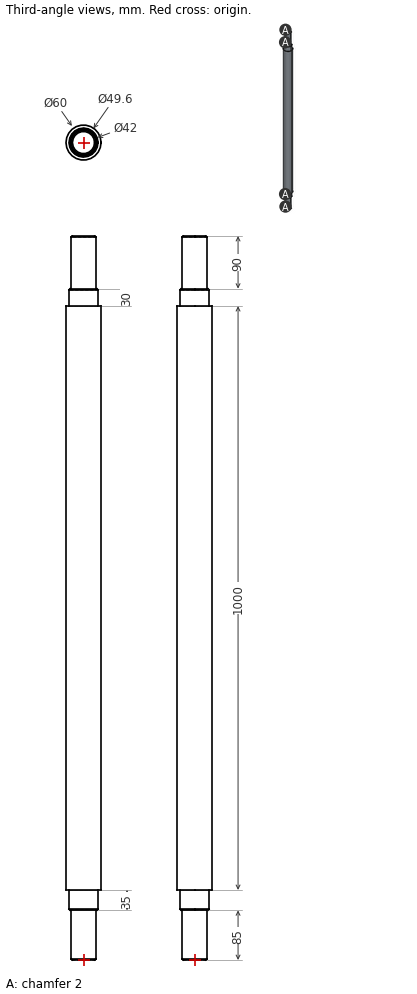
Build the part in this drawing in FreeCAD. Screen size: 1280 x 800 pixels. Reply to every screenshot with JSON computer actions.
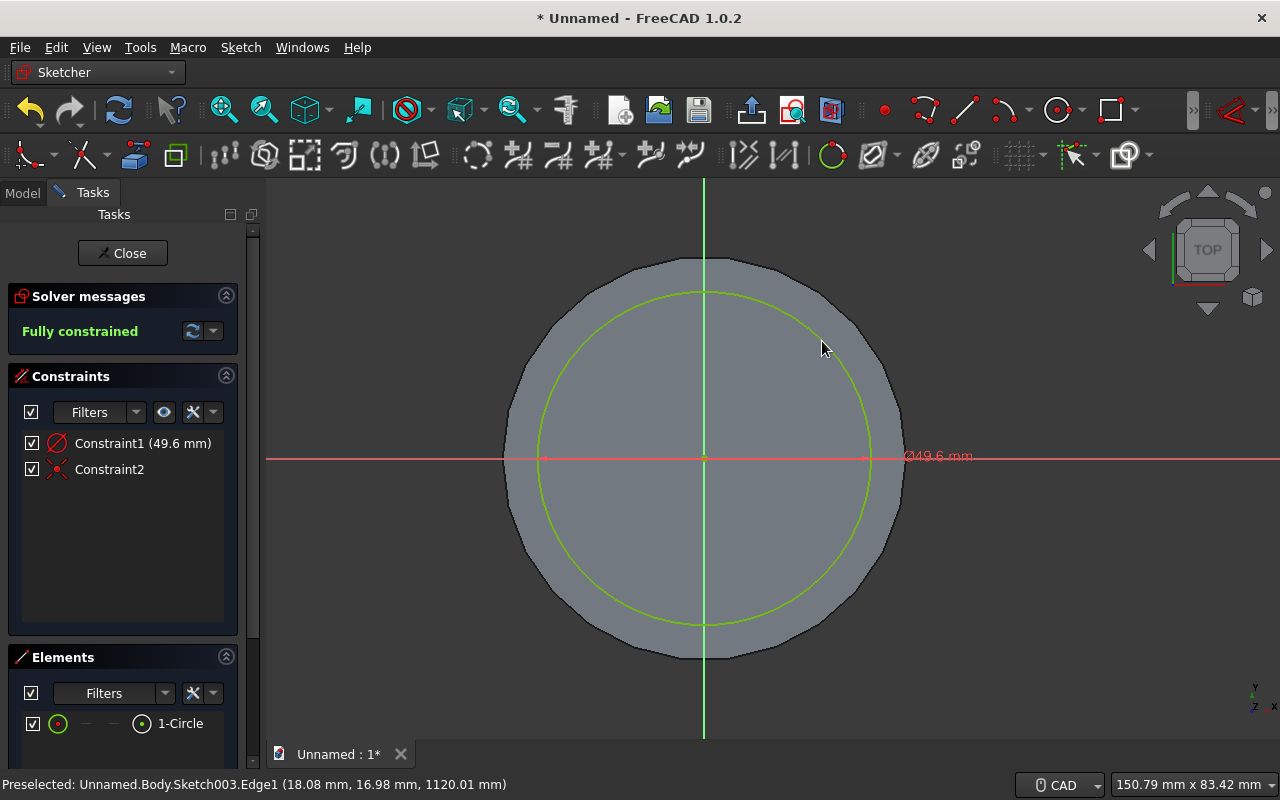
{"action": "left_click", "coordinate": [123, 253]}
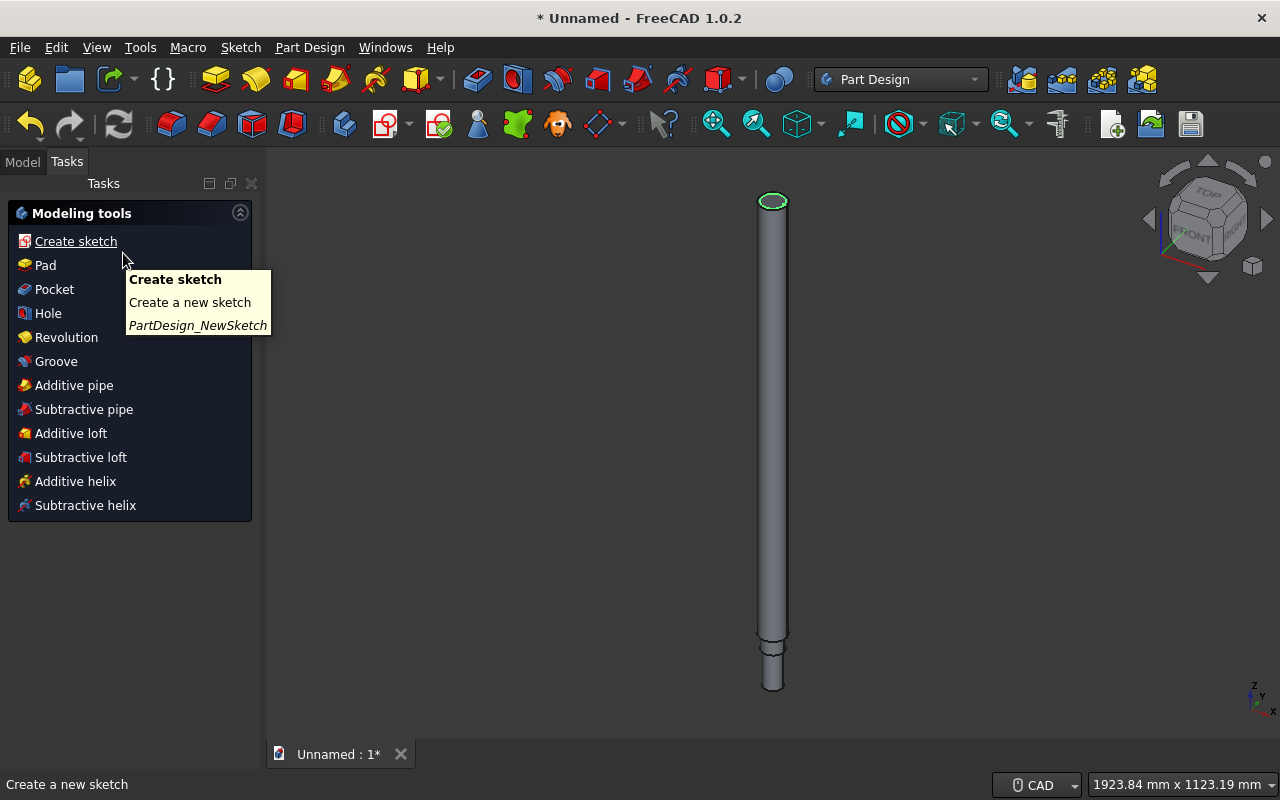
{"action": "left_click", "coordinate": [216, 80]}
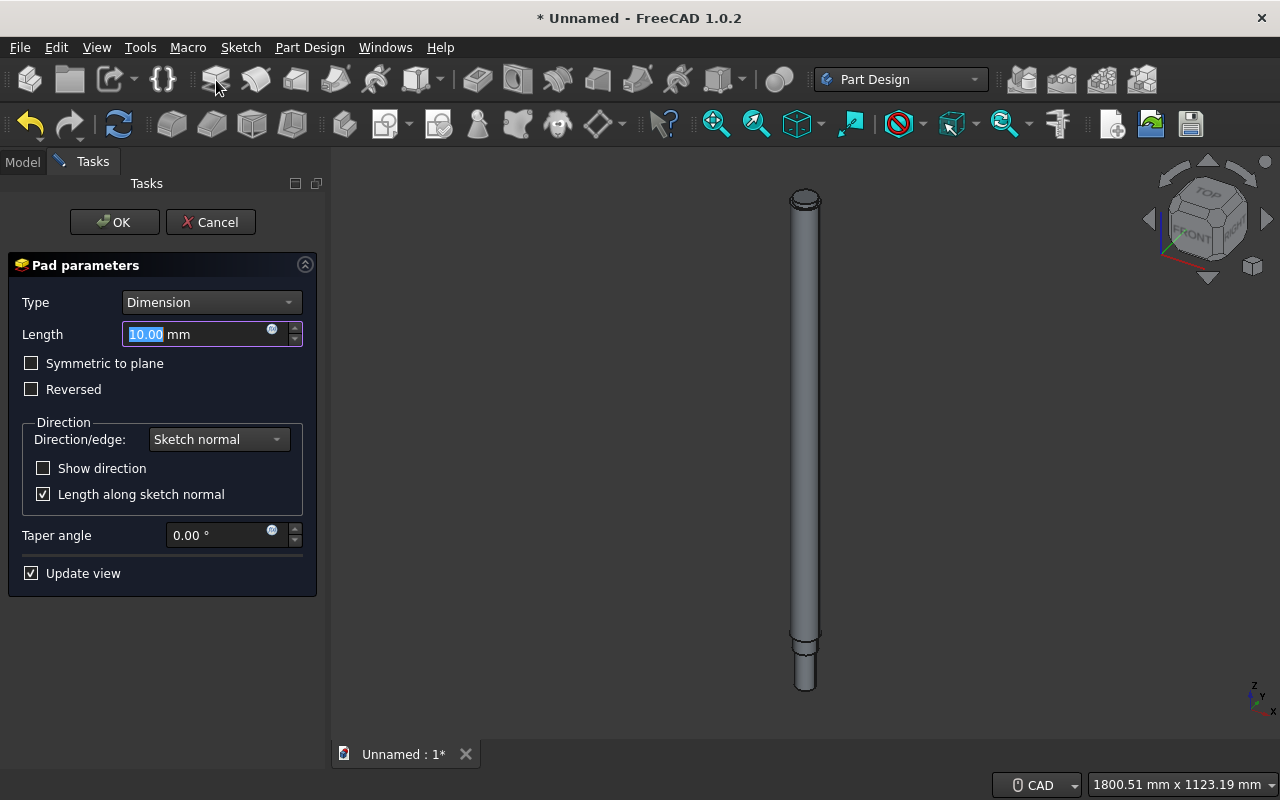
{"action": "type", "text": "30"}
{"action": "key", "text": "Tab"}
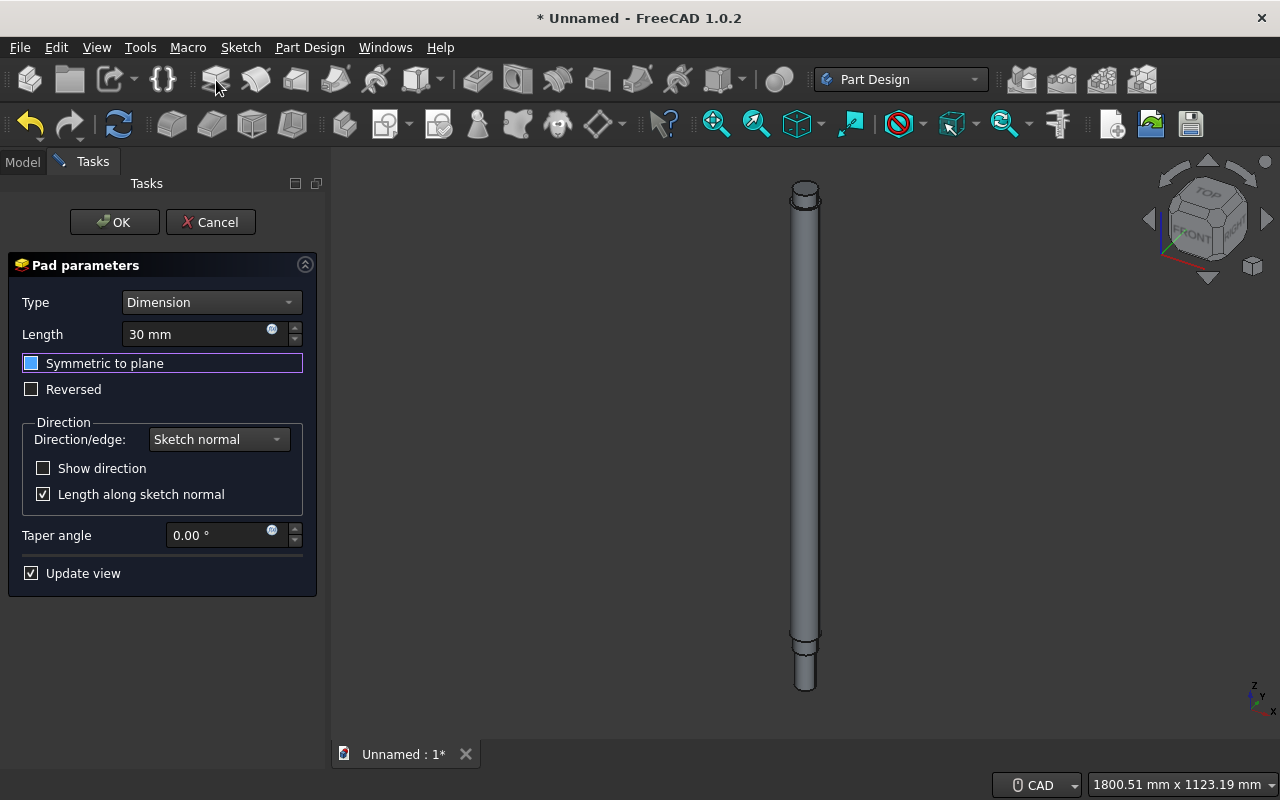
{"action": "left_click", "coordinate": [115, 222]}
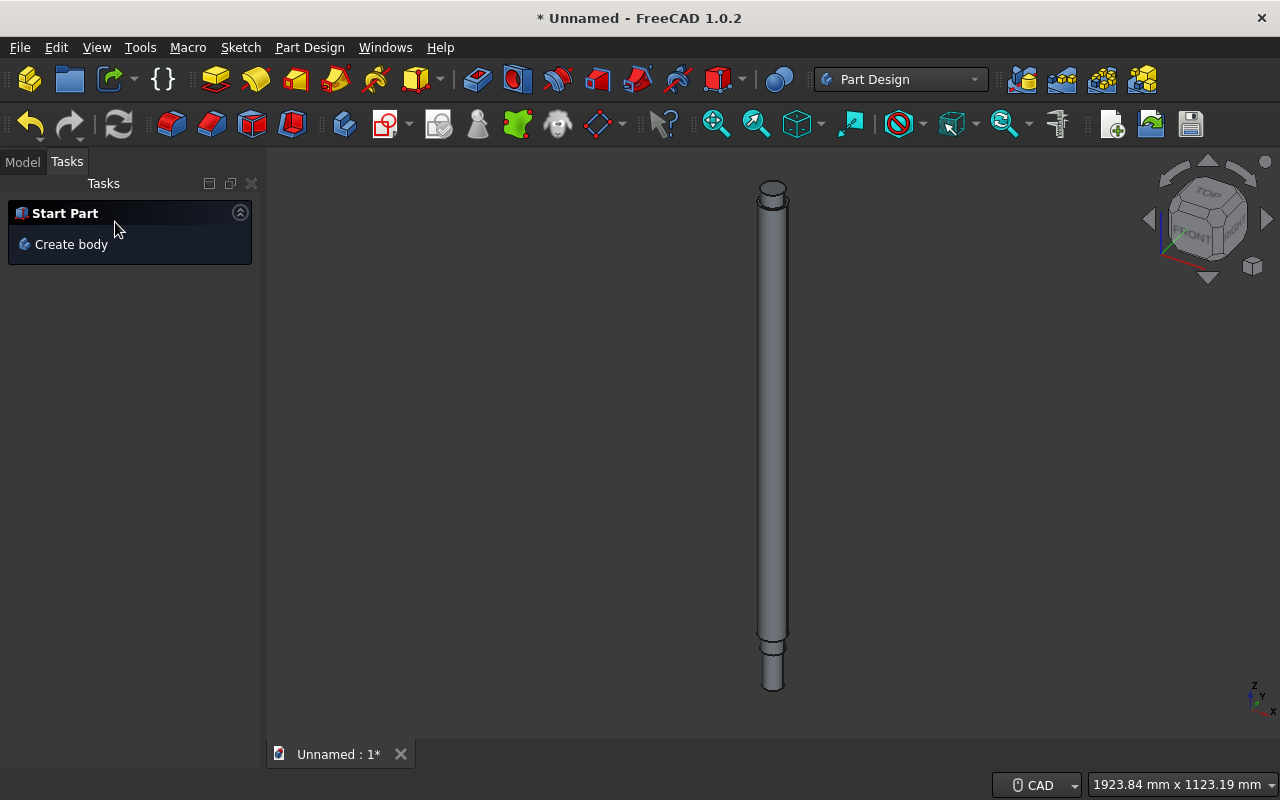
{"action": "left_click", "coordinate": [775, 185]}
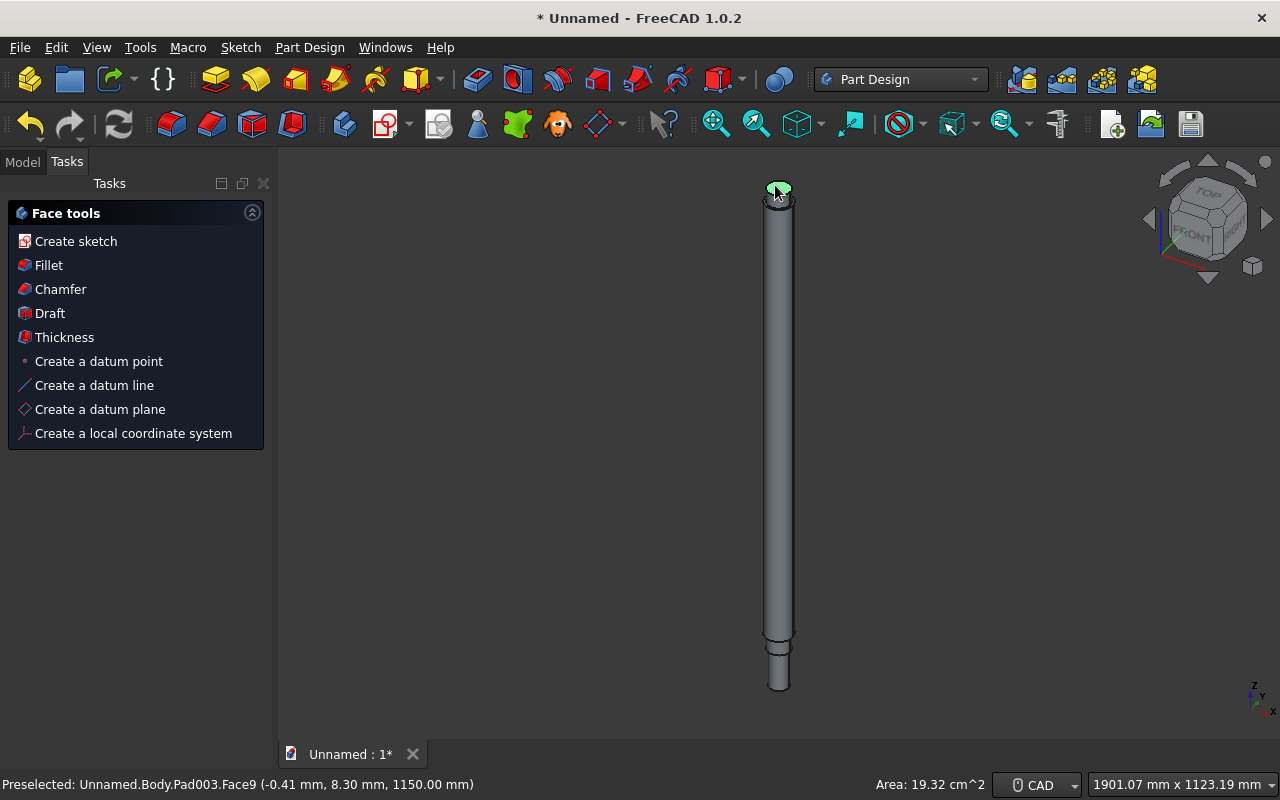
{"action": "left_click", "coordinate": [386, 124]}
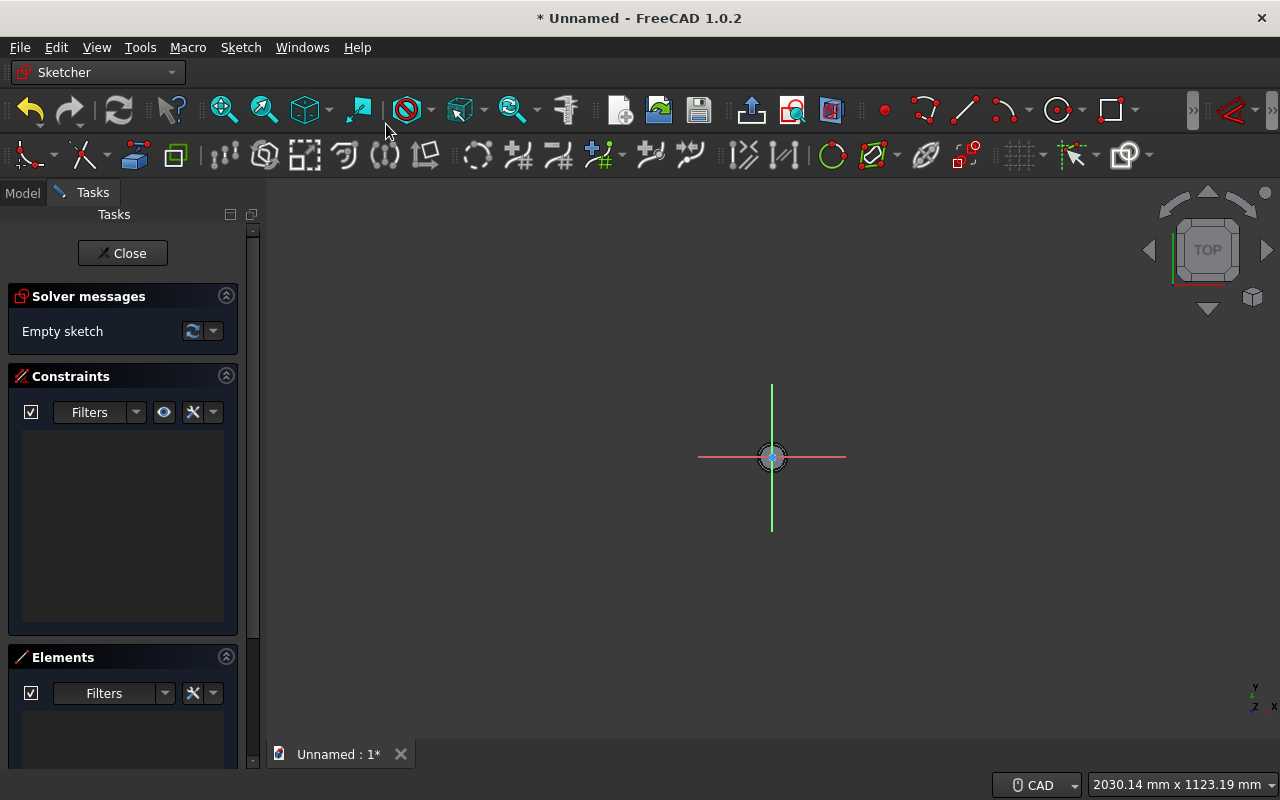
{"action": "scroll", "coordinate": [777, 457], "scroll_direction": "up", "scroll_amount": 14}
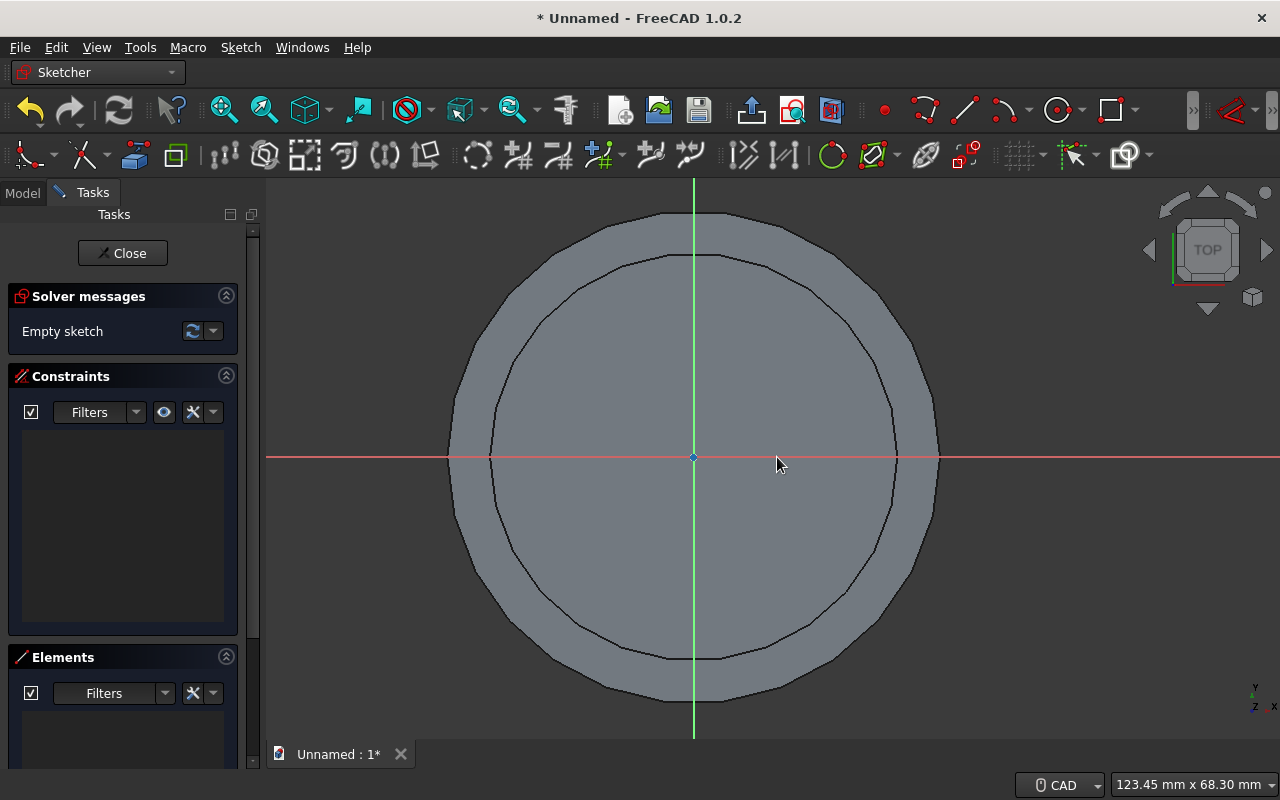
{"action": "key", "text": "g c"}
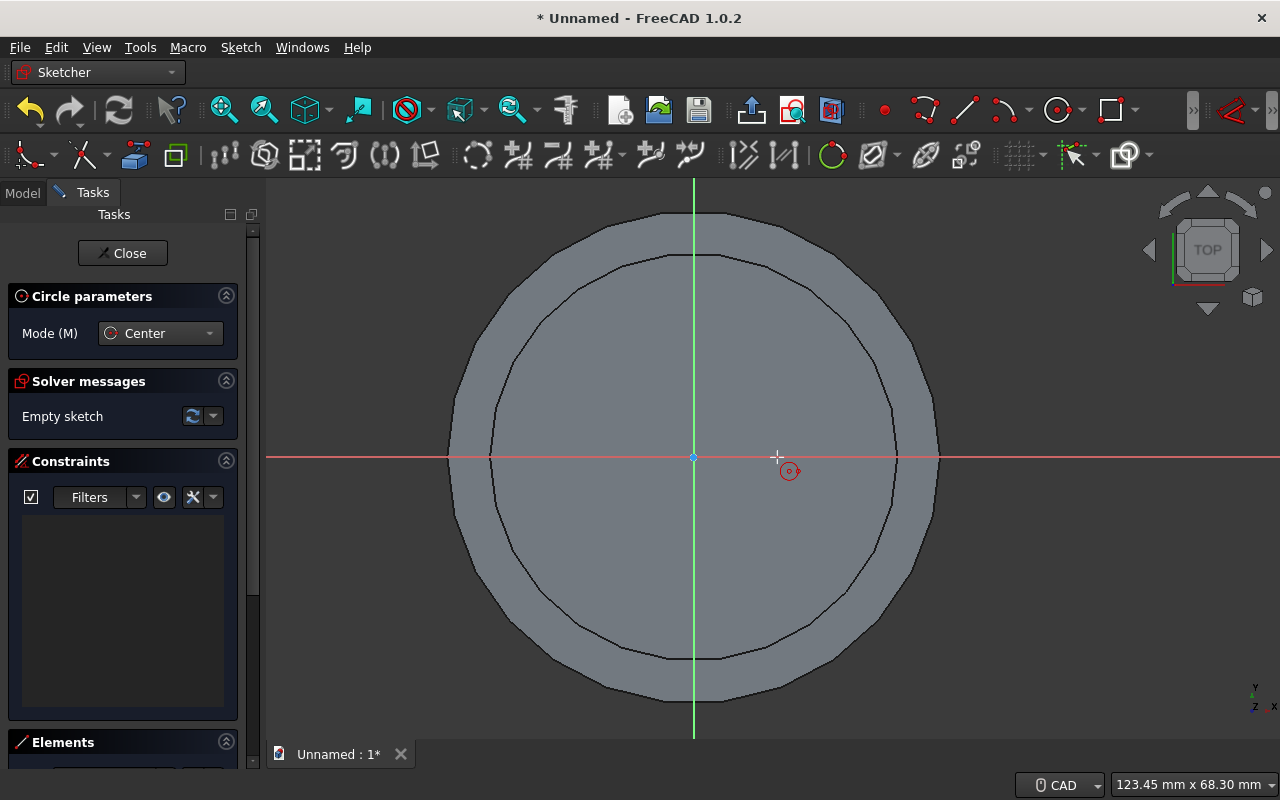
{"action": "left_click", "coordinate": [694, 457]}
{"action": "mouse_move", "coordinate": [816, 335]}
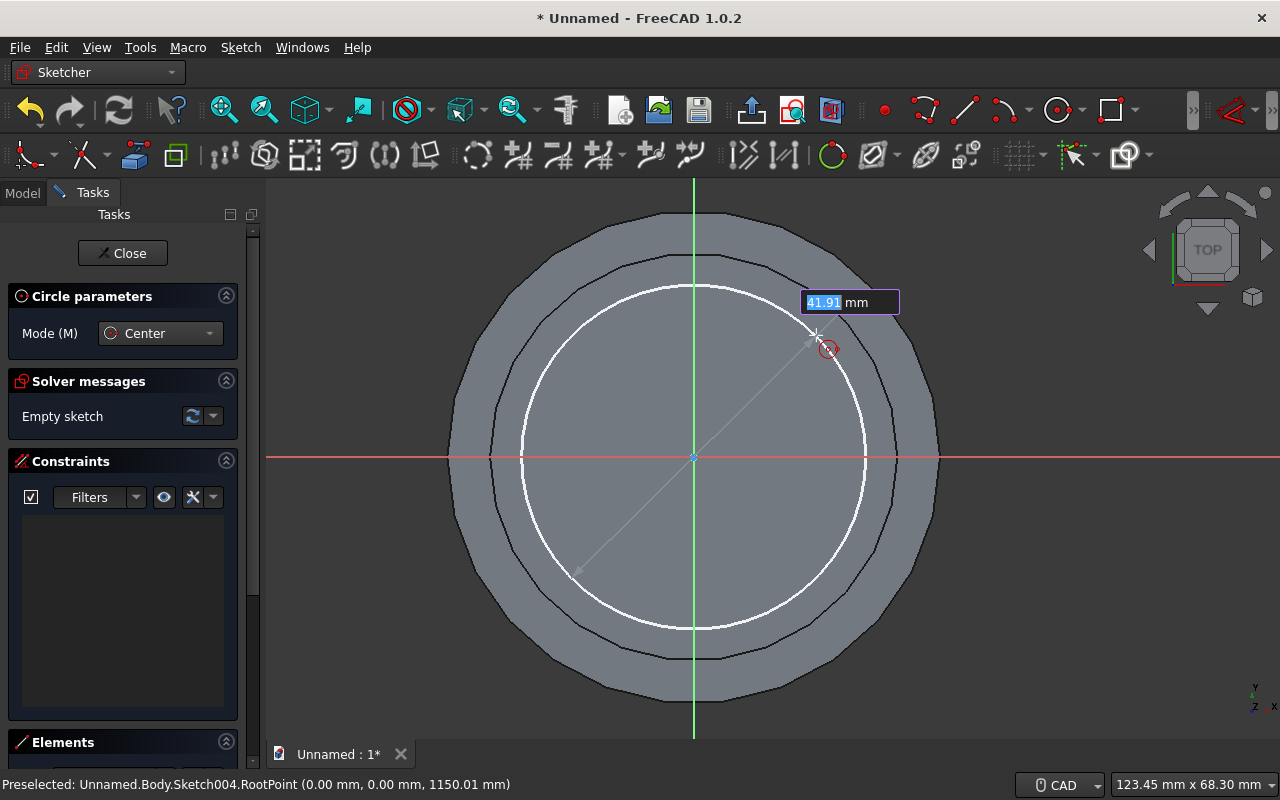
{"action": "type", "text": "42"}
{"action": "key", "text": "Return"}
{"action": "key", "text": "Escape"}